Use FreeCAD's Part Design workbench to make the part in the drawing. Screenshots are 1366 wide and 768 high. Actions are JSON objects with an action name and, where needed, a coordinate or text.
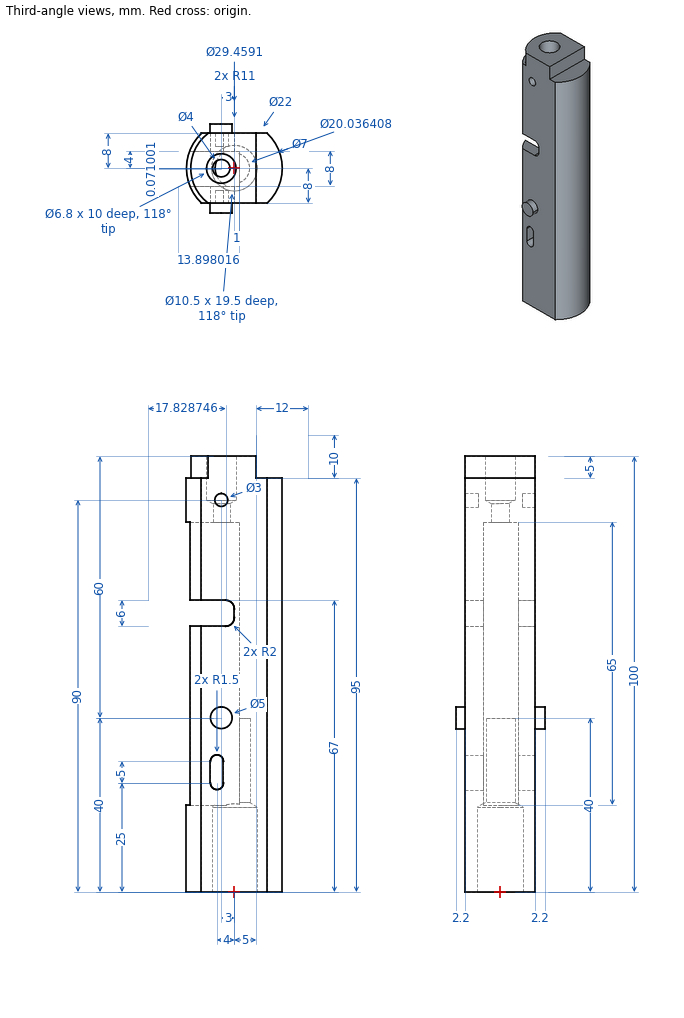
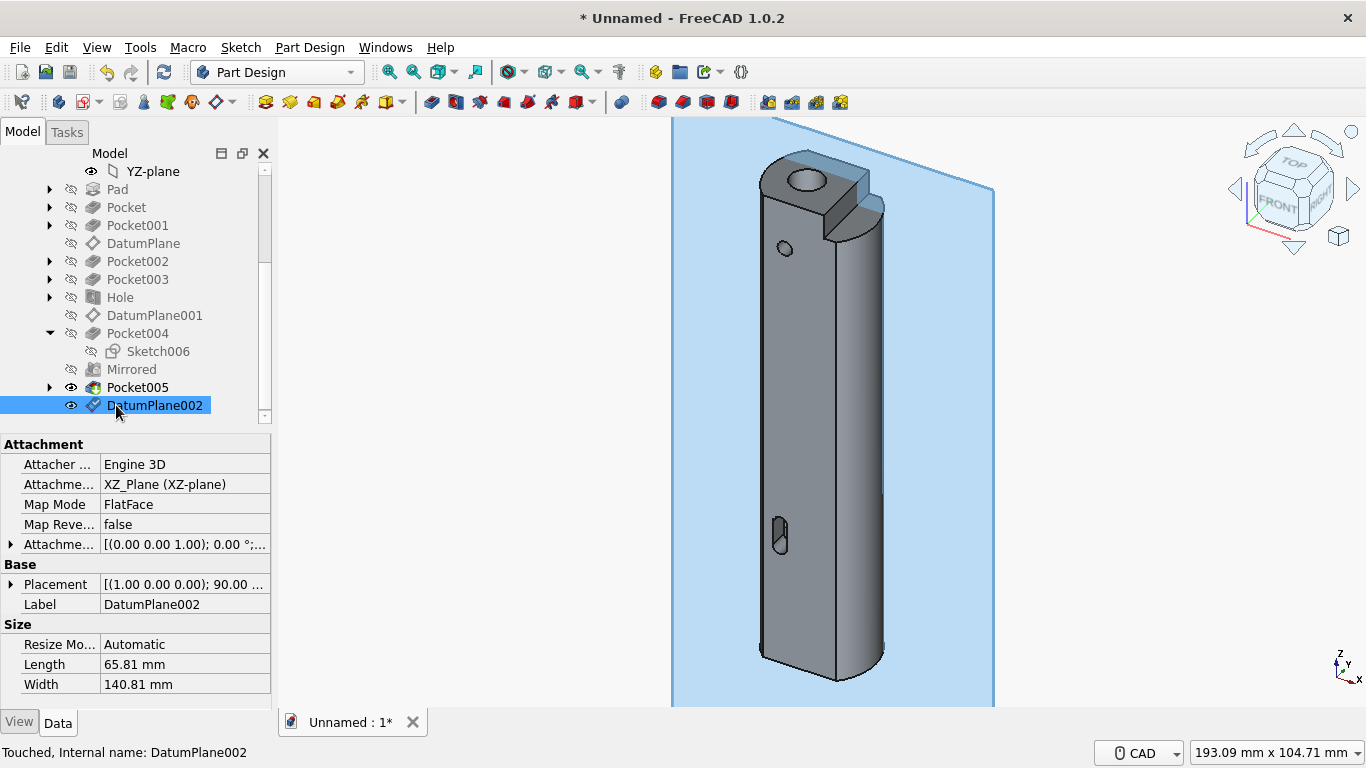
{"action": "left_click", "coordinate": [84, 102]}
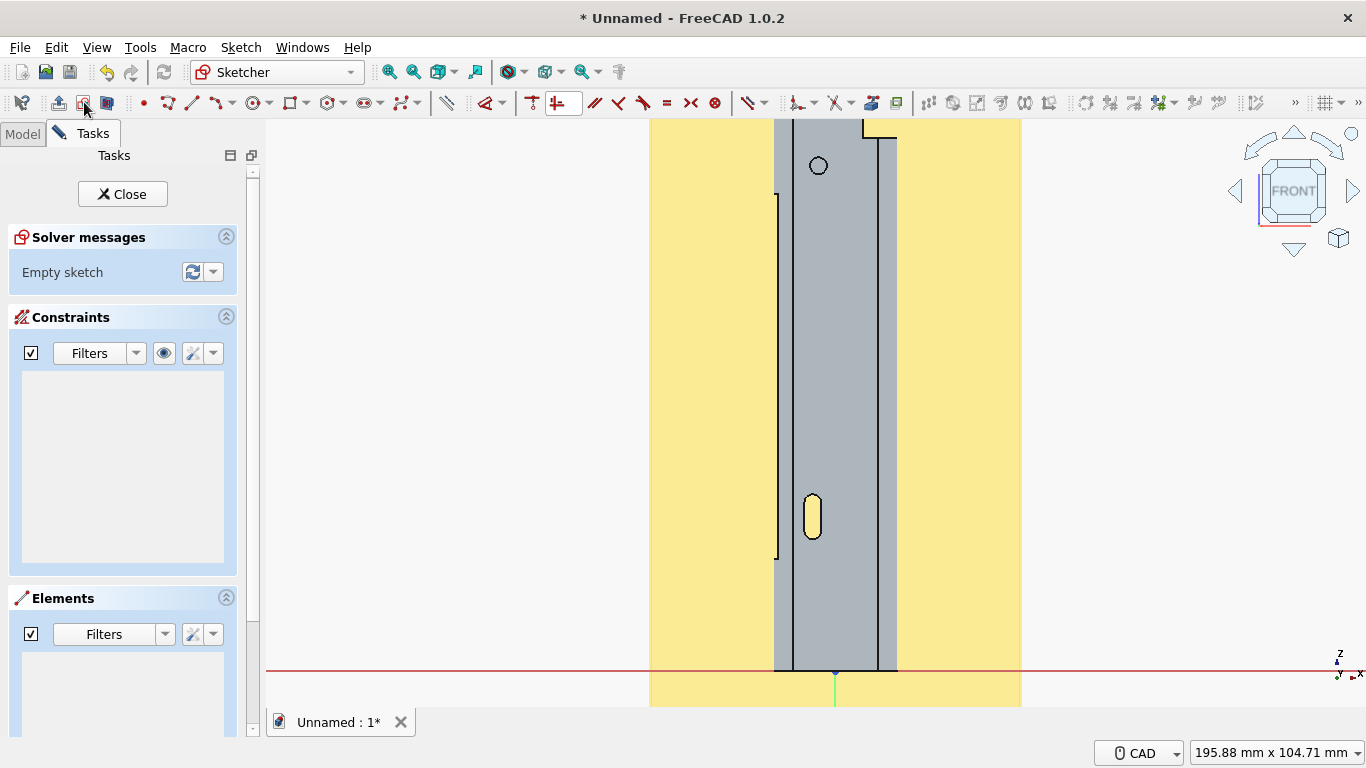
{"action": "key", "text": "q s"}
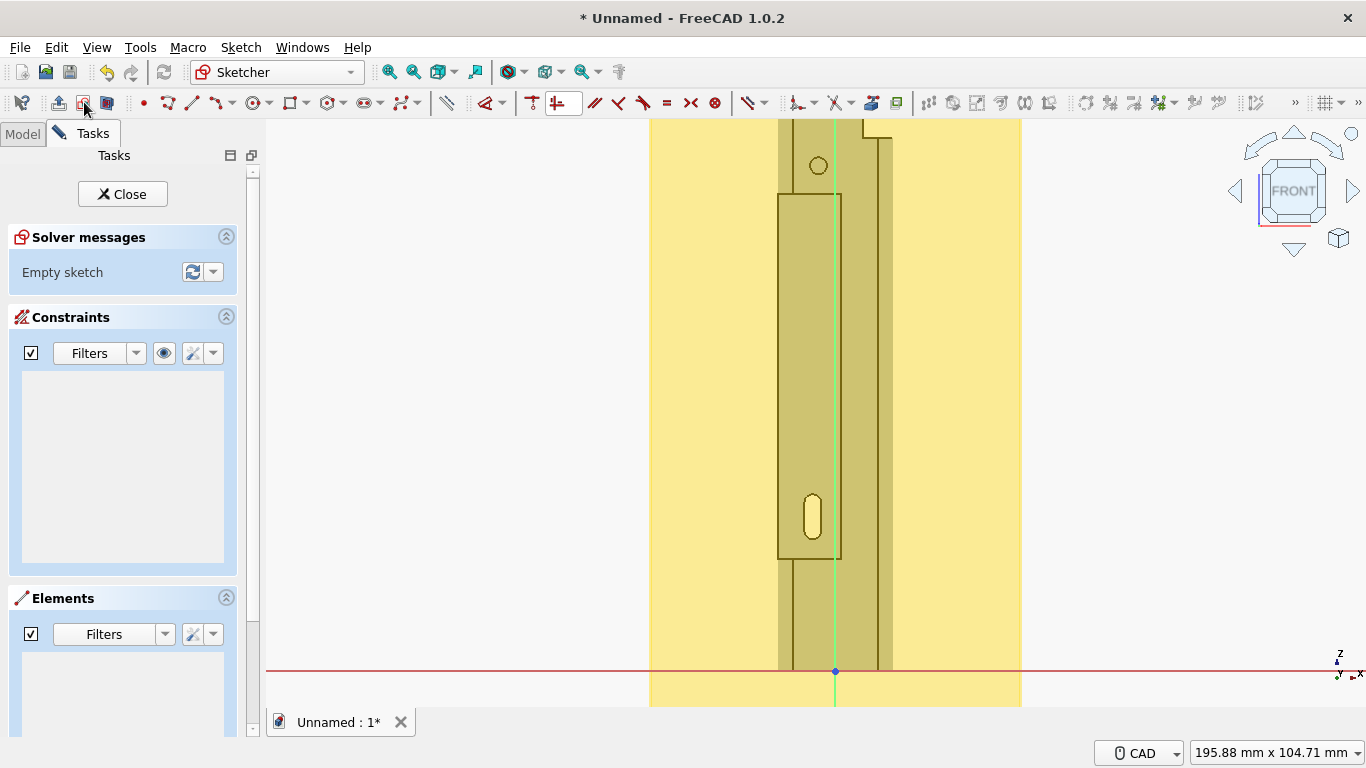
{"action": "scroll", "coordinate": [786, 292], "scroll_direction": "up", "scroll_amount": 9}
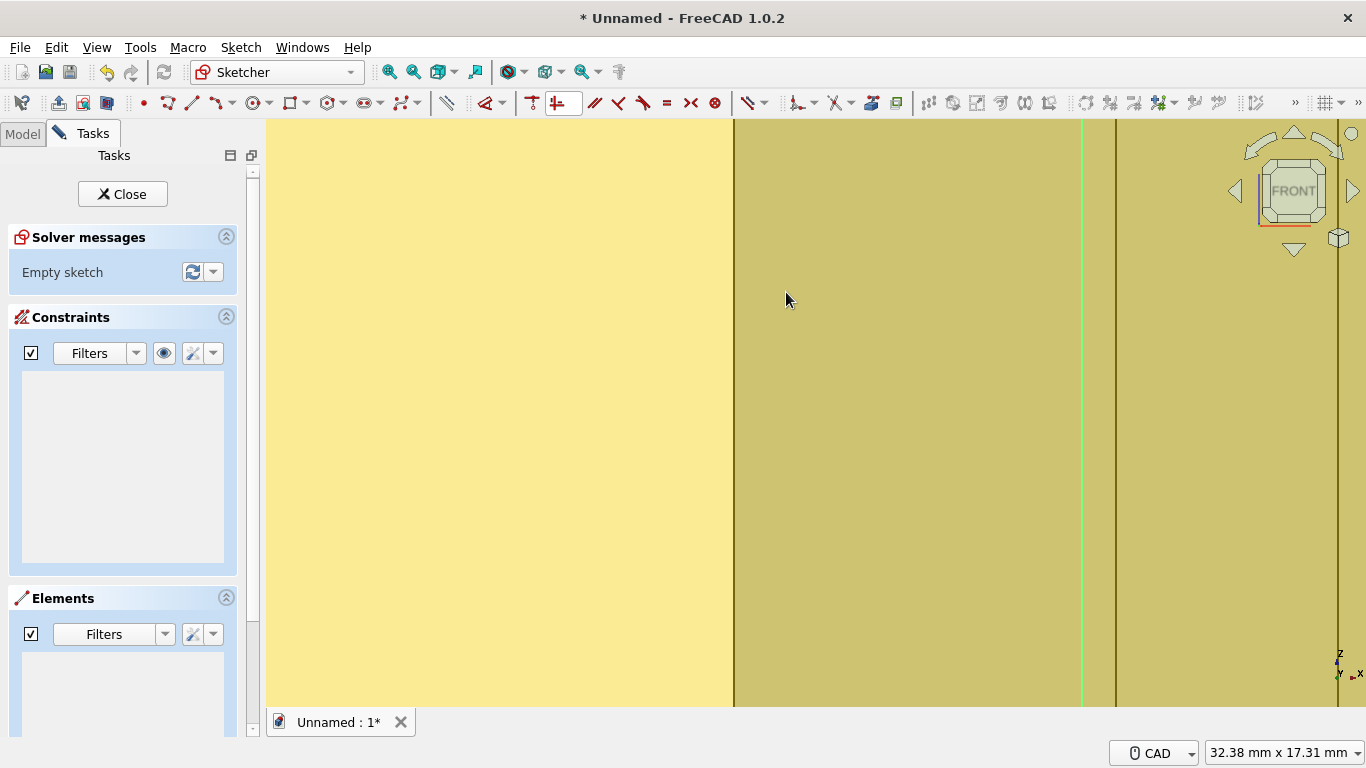
{"action": "left_click", "coordinate": [168, 104]}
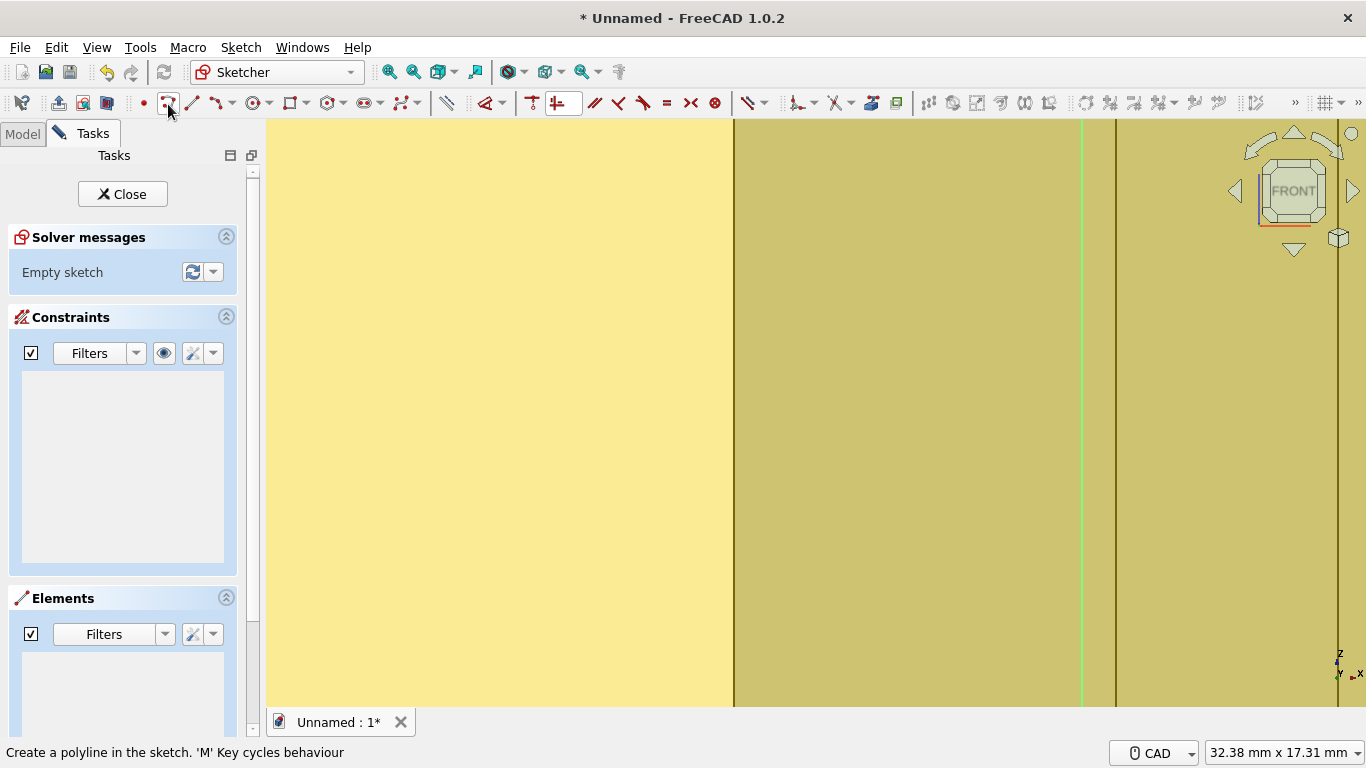
{"action": "left_click", "coordinate": [1014, 309]}
{"action": "left_click", "coordinate": [408, 309]}
{"action": "left_click", "coordinate": [408, 512]}
{"action": "left_click", "coordinate": [1014, 512]}
{"action": "right_click", "coordinate": [1014, 512]}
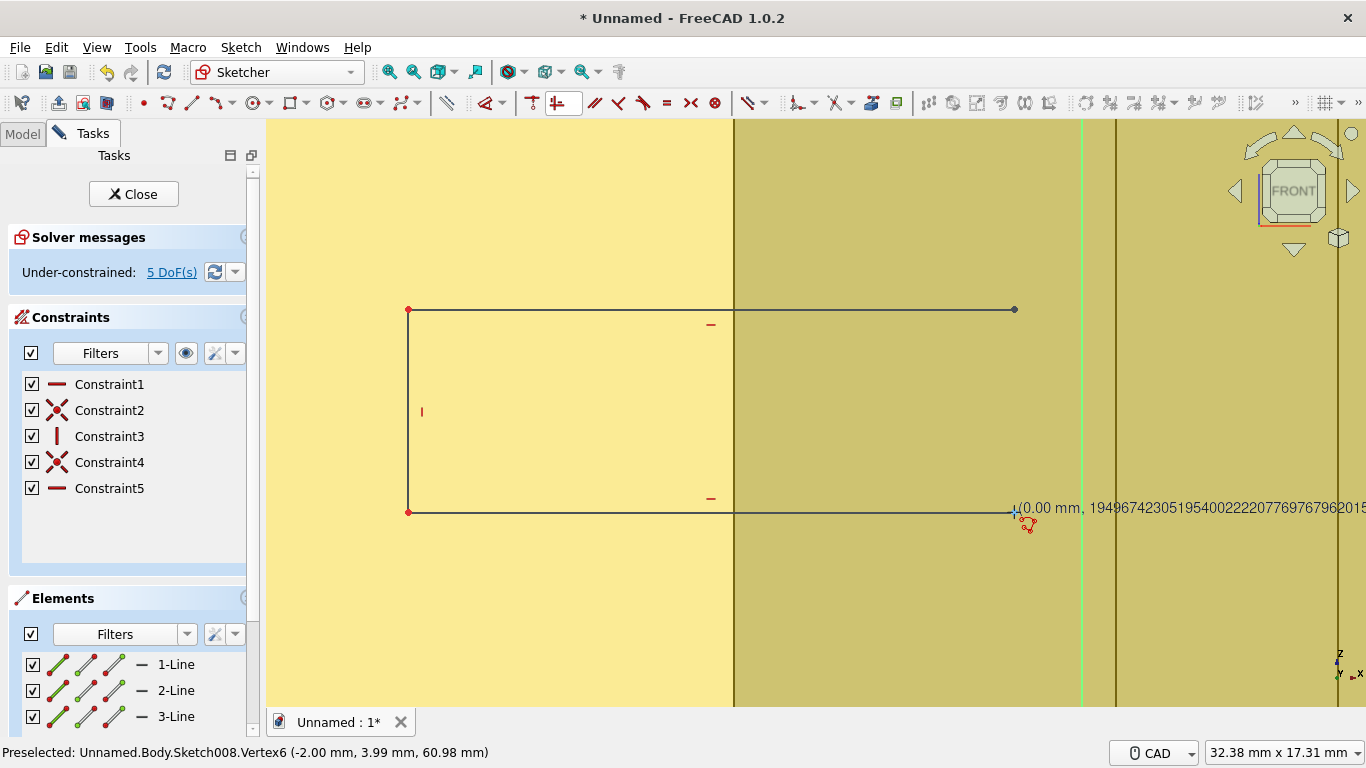
{"action": "key", "text": "g l"}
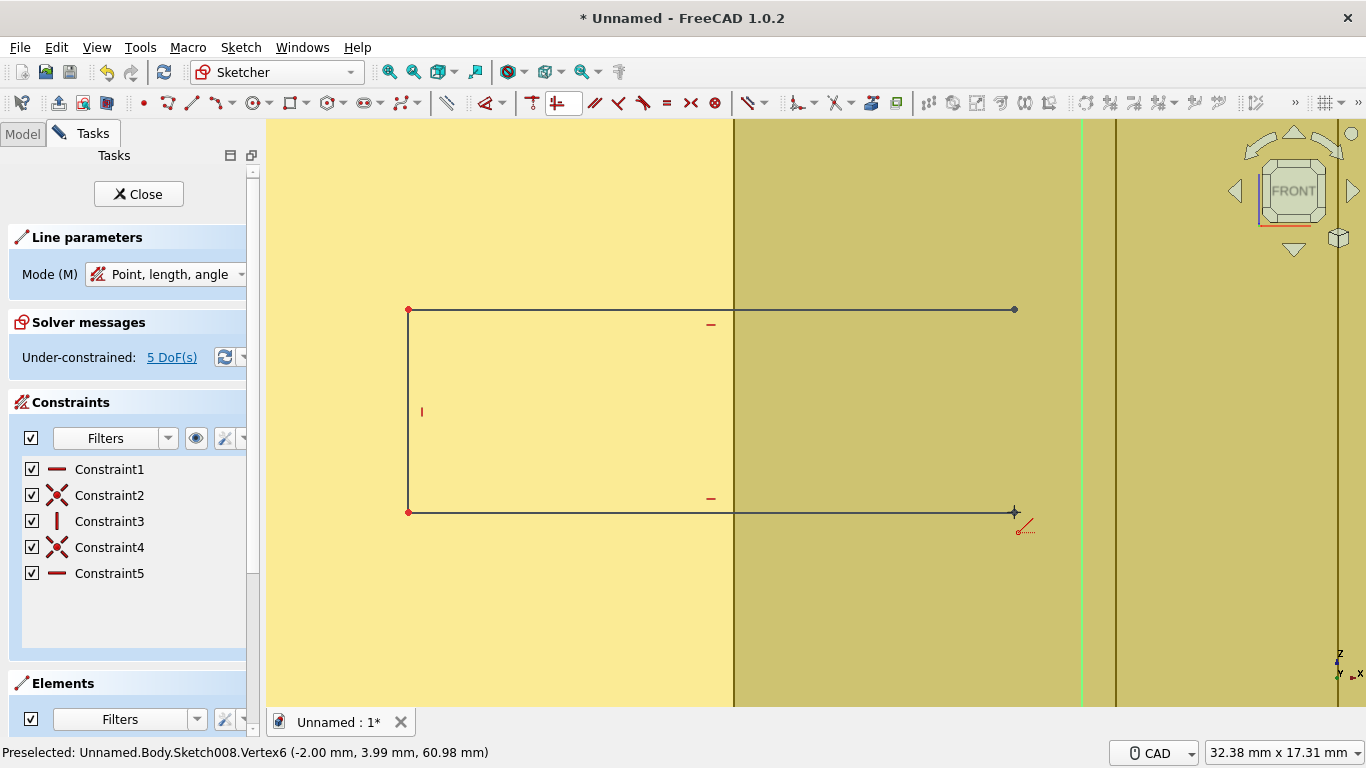
{"action": "left_click", "coordinate": [1082, 444]}
{"action": "left_click", "coordinate": [1073, 376]}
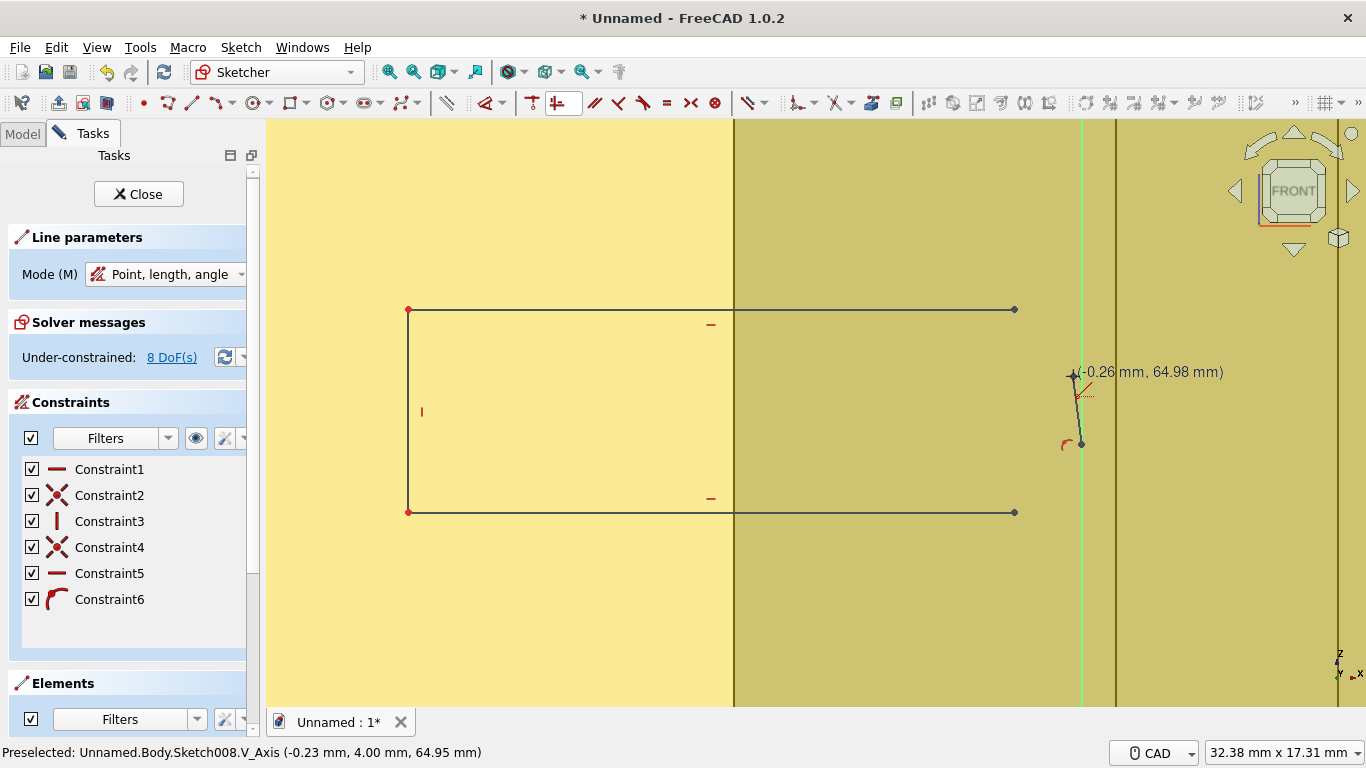
{"action": "left_click", "coordinate": [216, 104]}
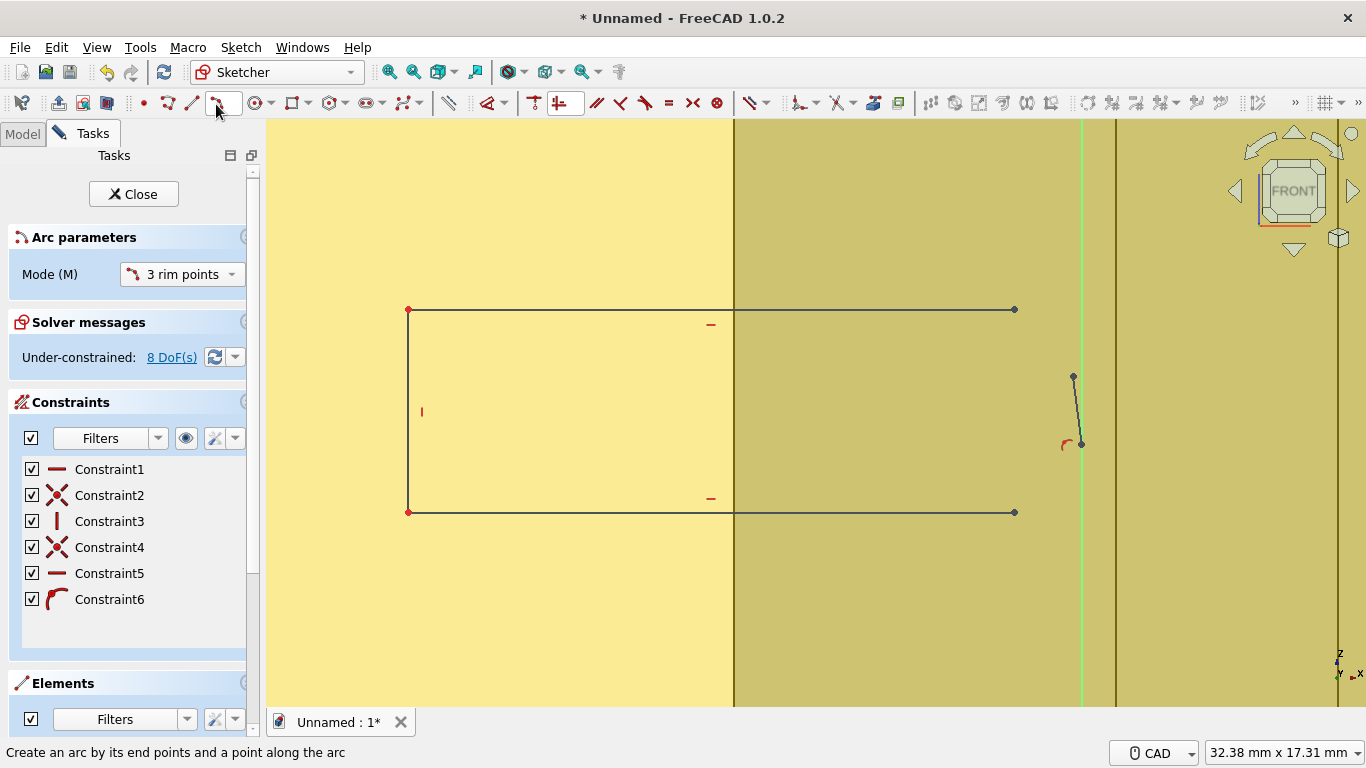
{"action": "left_click", "coordinate": [1014, 513]}
{"action": "left_click", "coordinate": [1082, 445]}
{"action": "left_click", "coordinate": [1062, 492]}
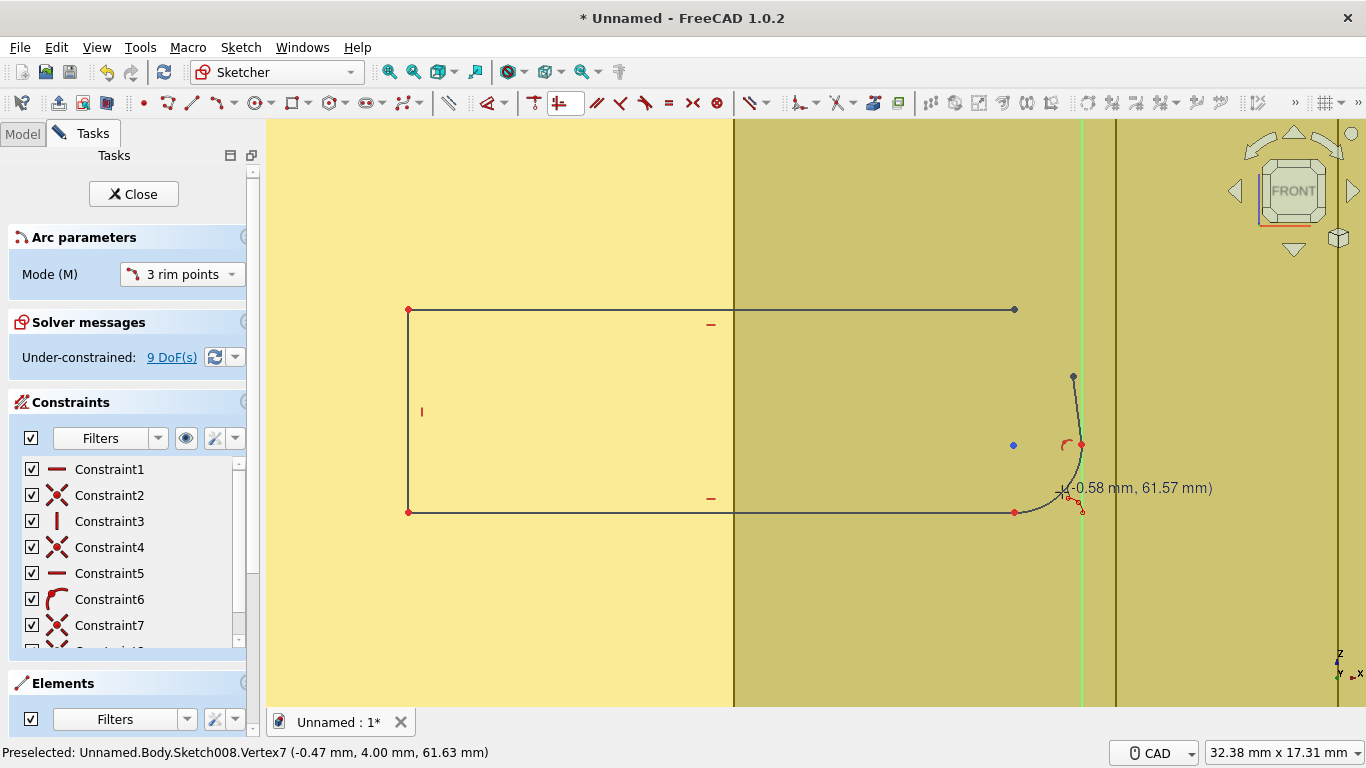
{"action": "left_click", "coordinate": [1073, 377]}
{"action": "left_click", "coordinate": [1014, 310]}
{"action": "left_click", "coordinate": [1062, 328]}
{"action": "key", "text": "Escape"}